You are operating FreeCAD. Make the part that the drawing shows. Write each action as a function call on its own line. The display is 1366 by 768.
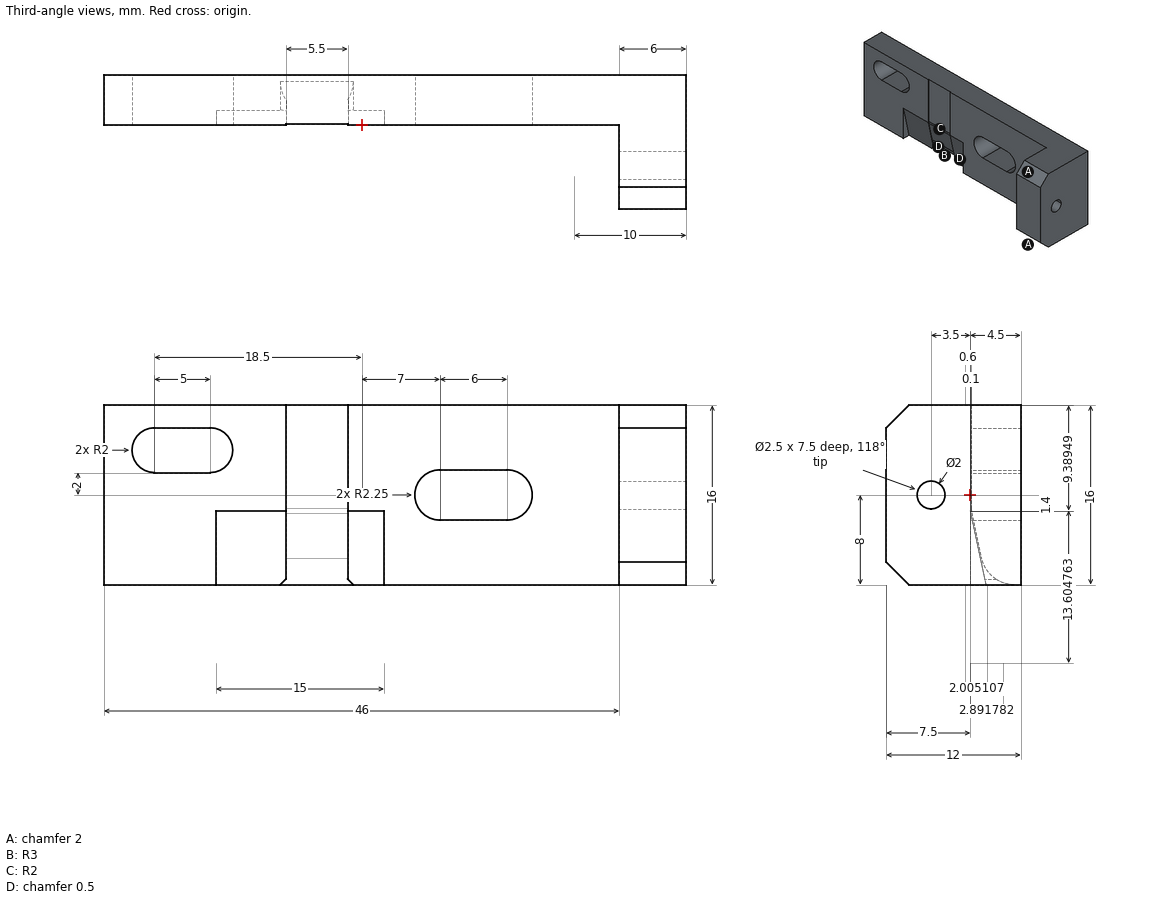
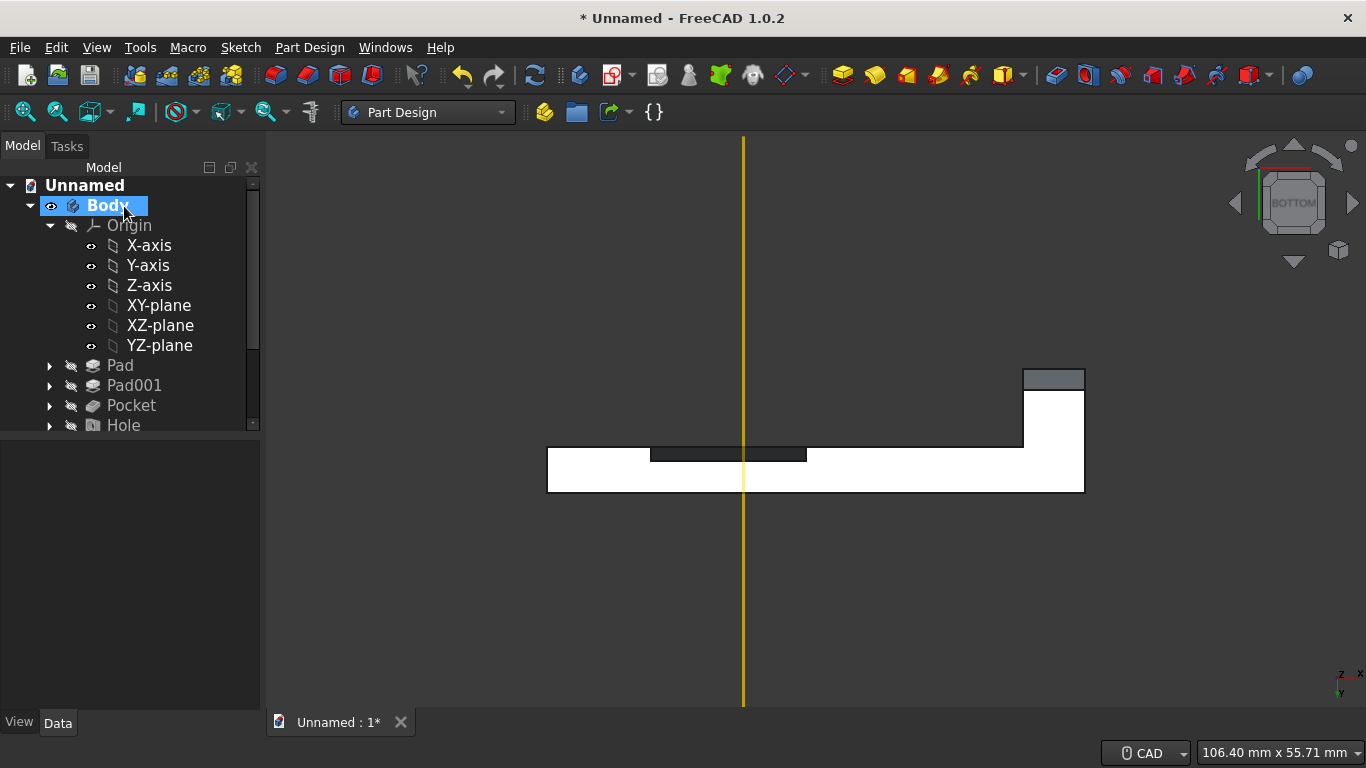
scroll(100, 301, down, 3)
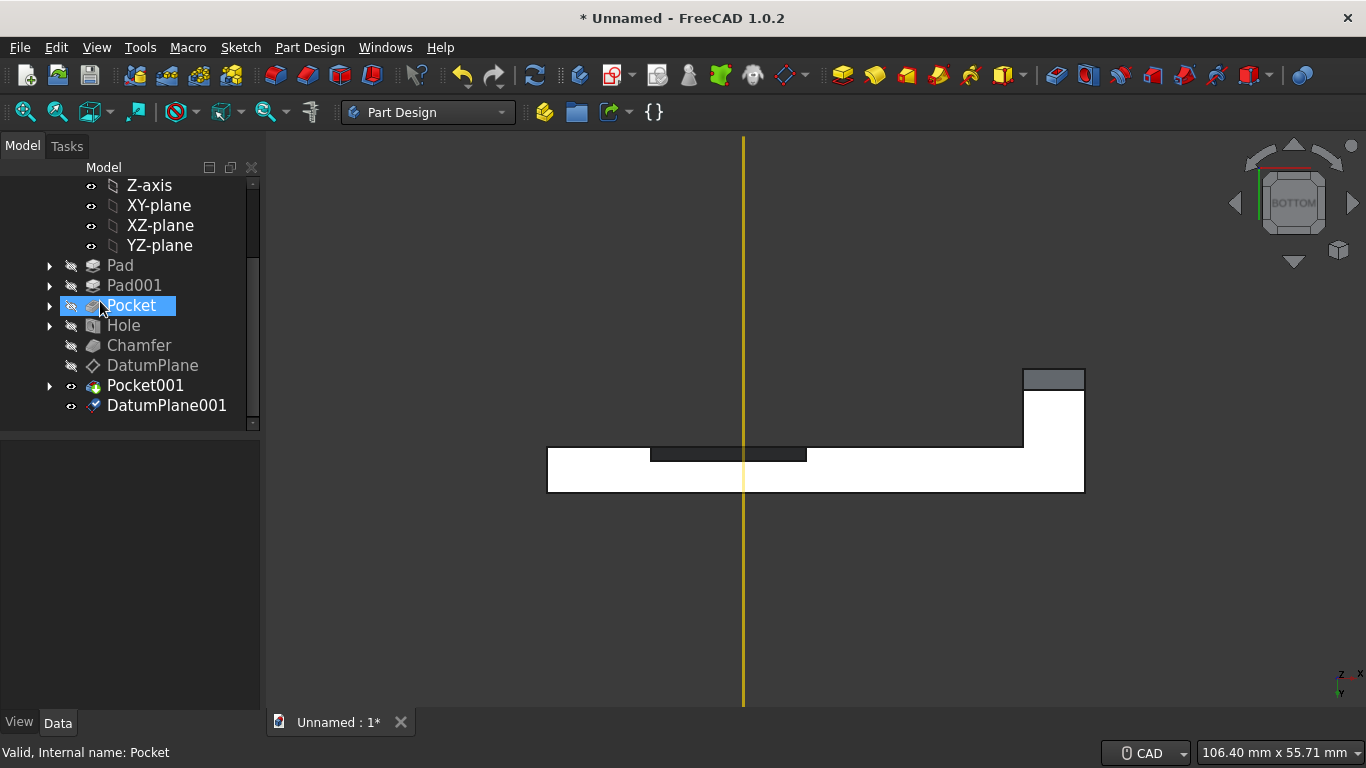
click(116, 406)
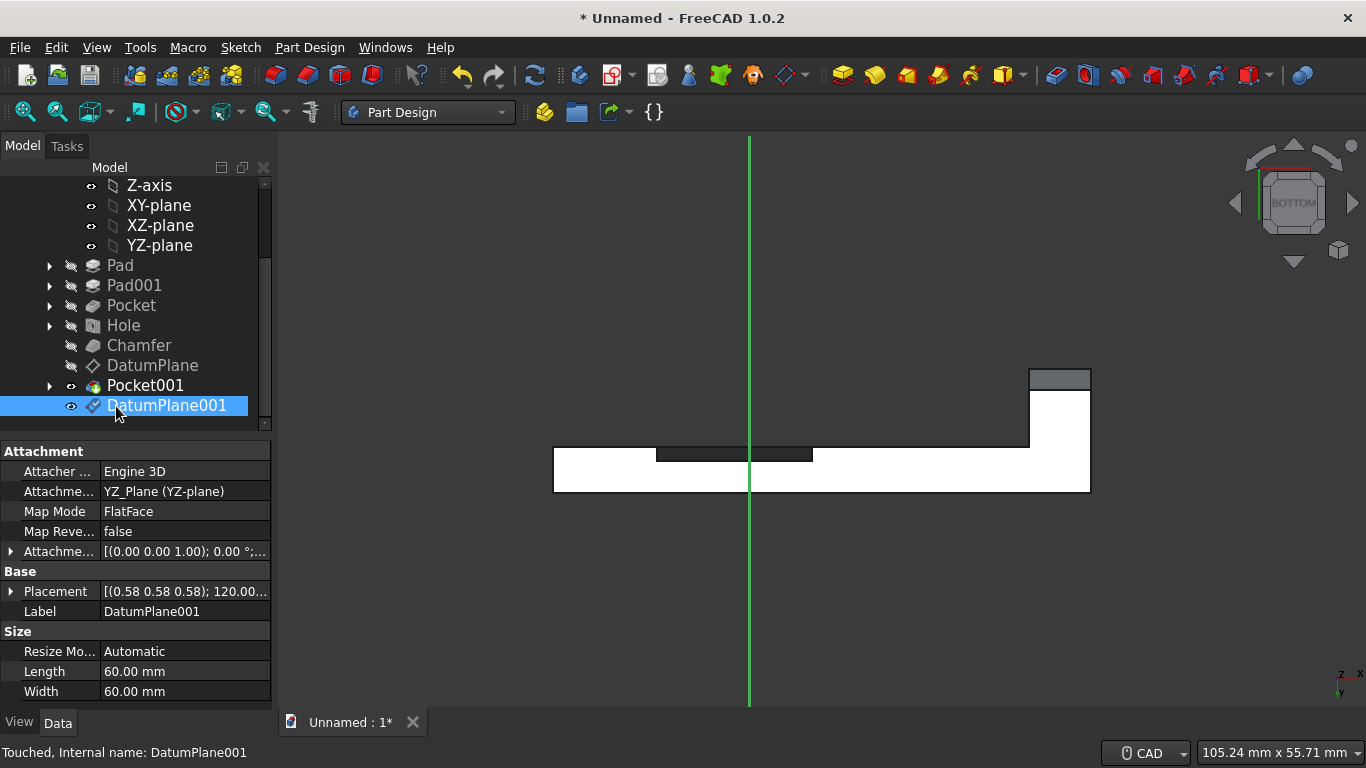
click(612, 76)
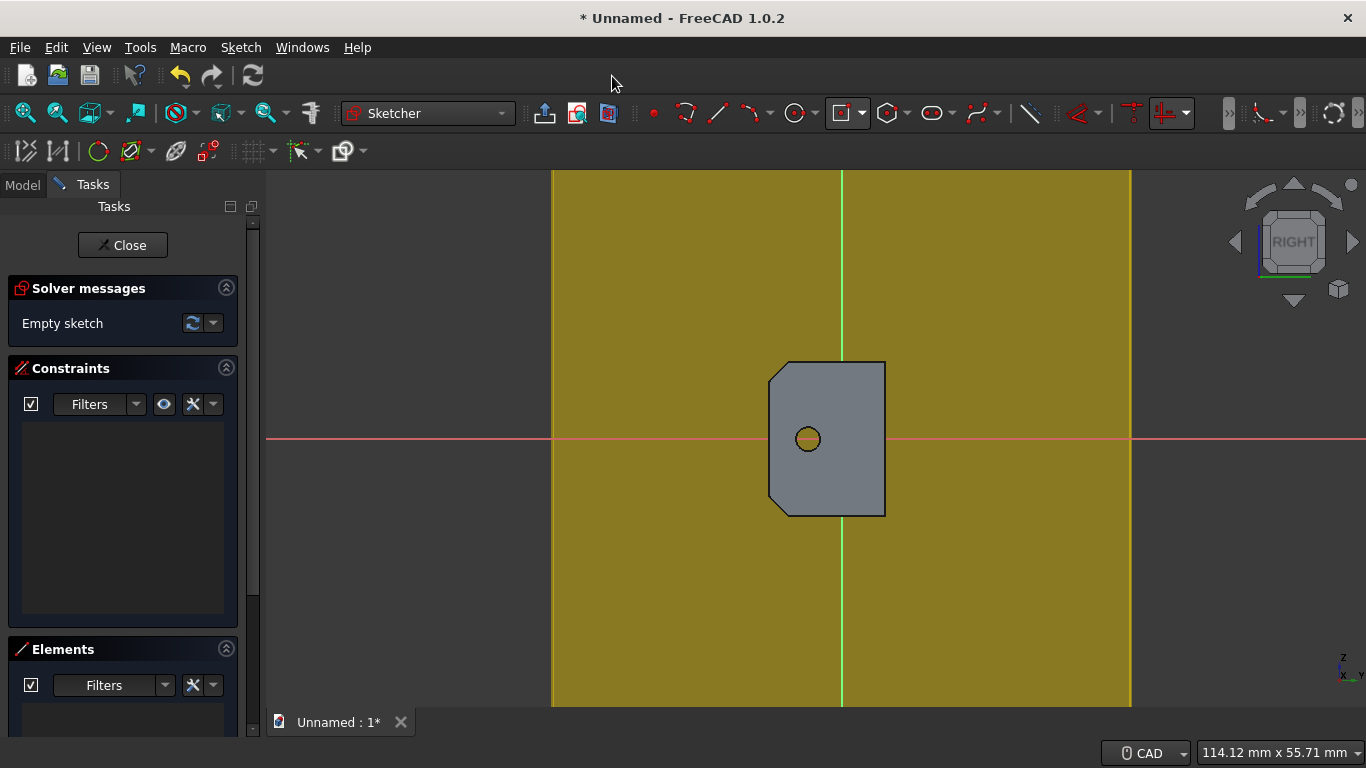
click(610, 114)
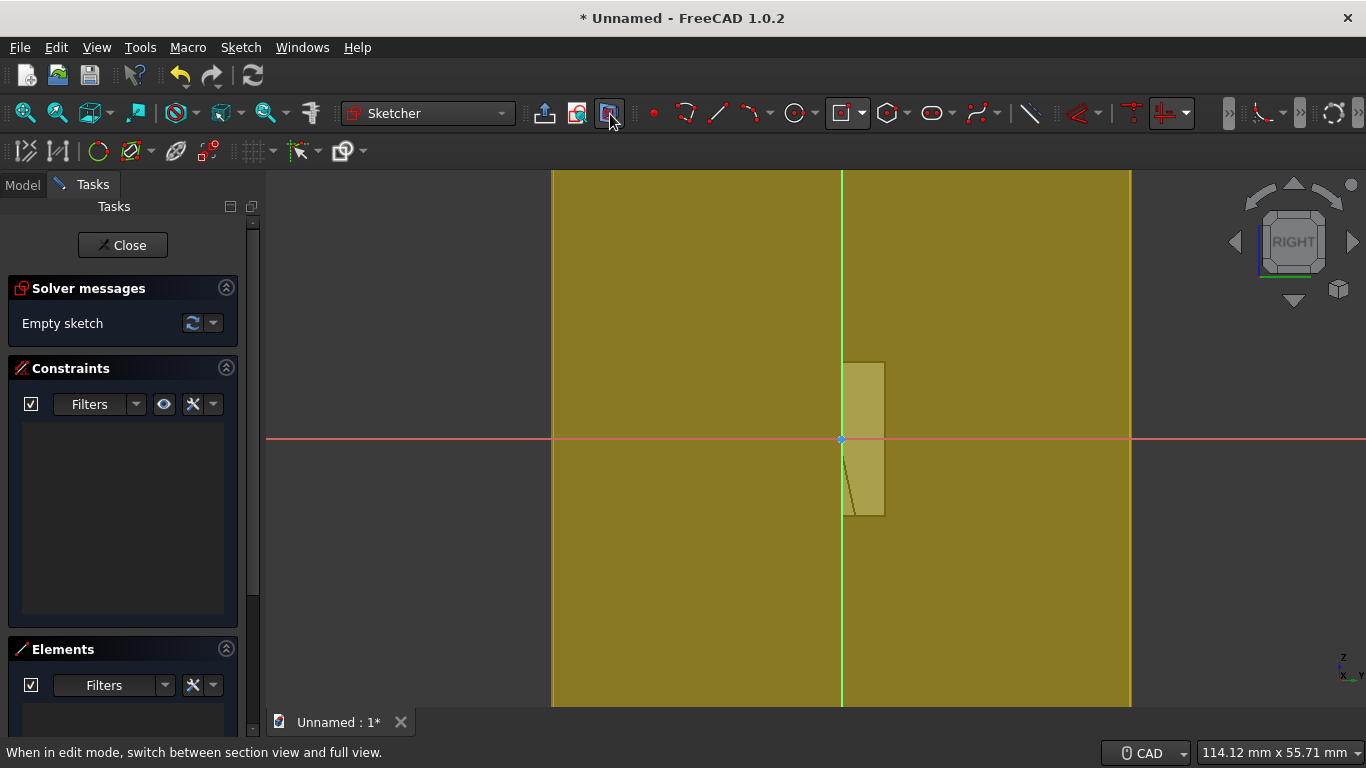
scroll(928, 440, up, 4)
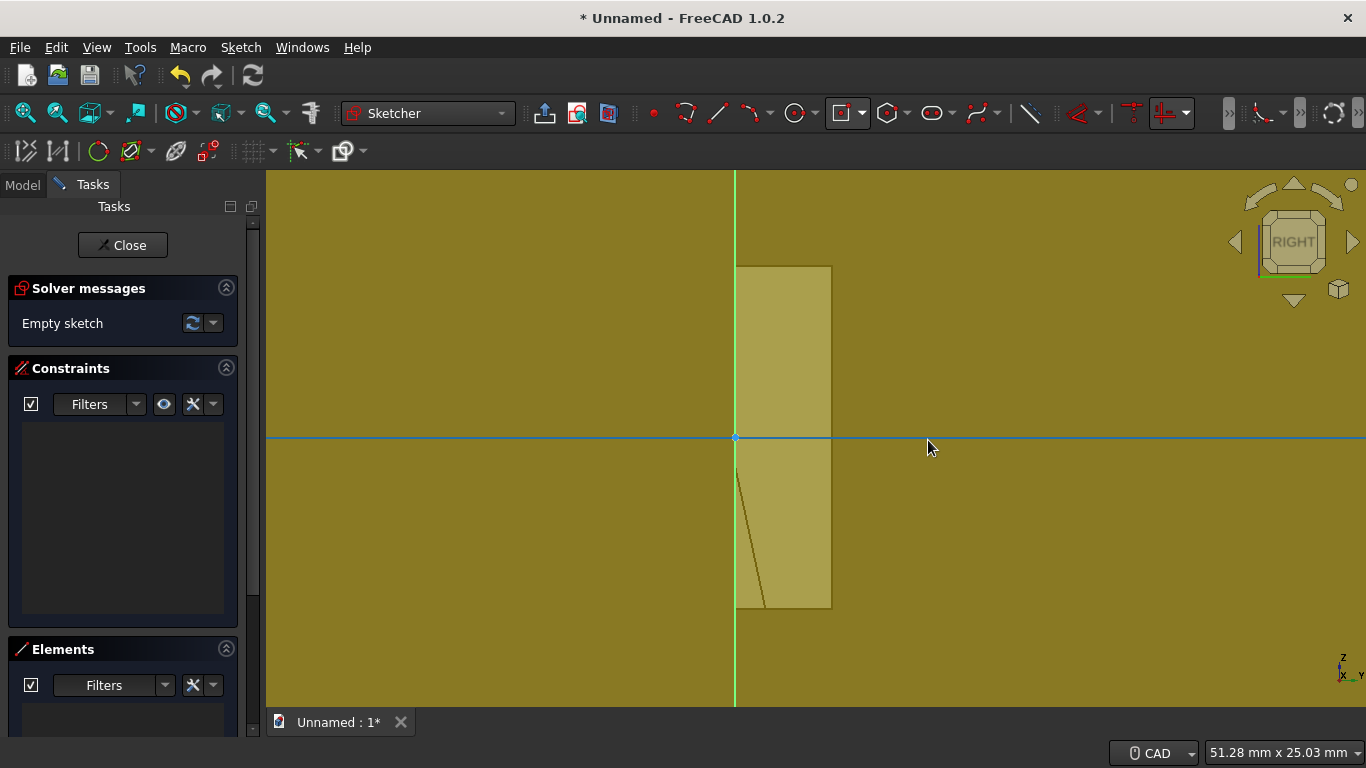
key(g)
key(m)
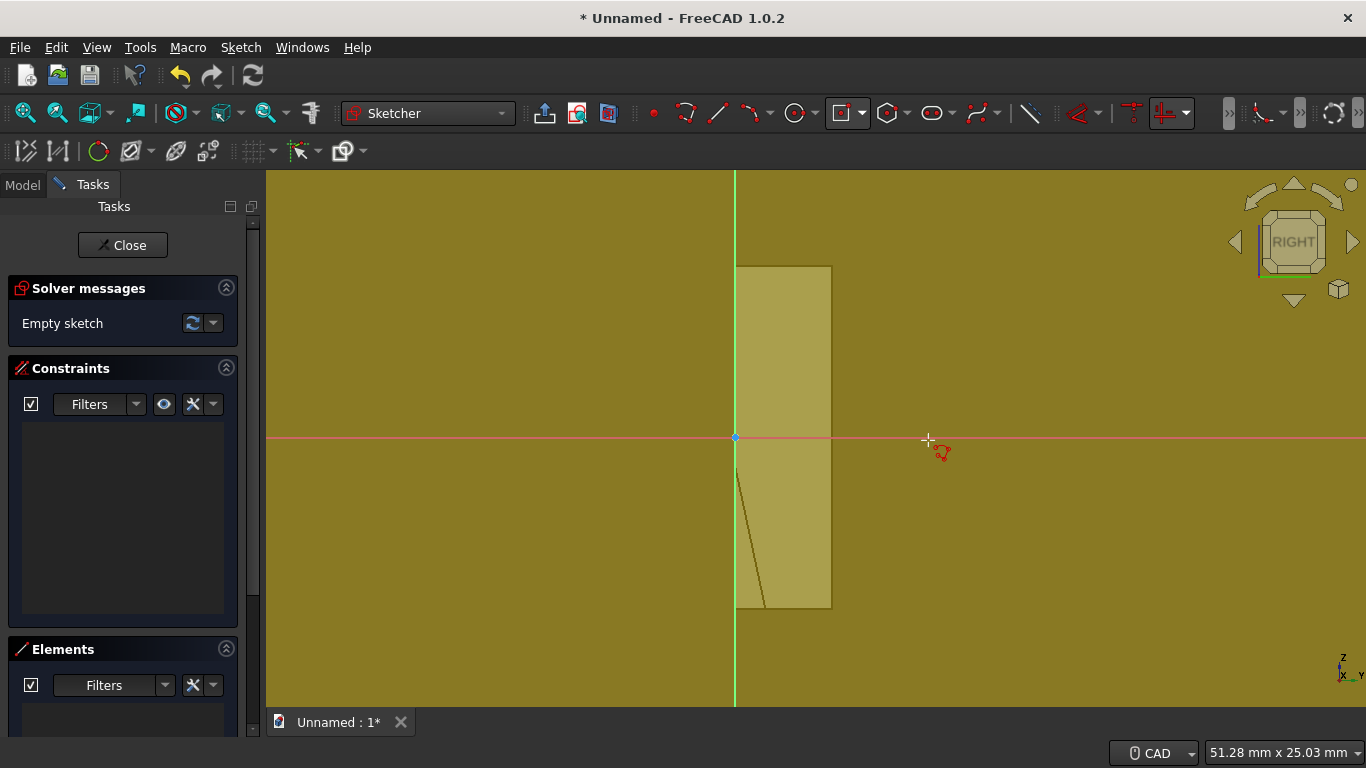
scroll(738, 467, up, 11)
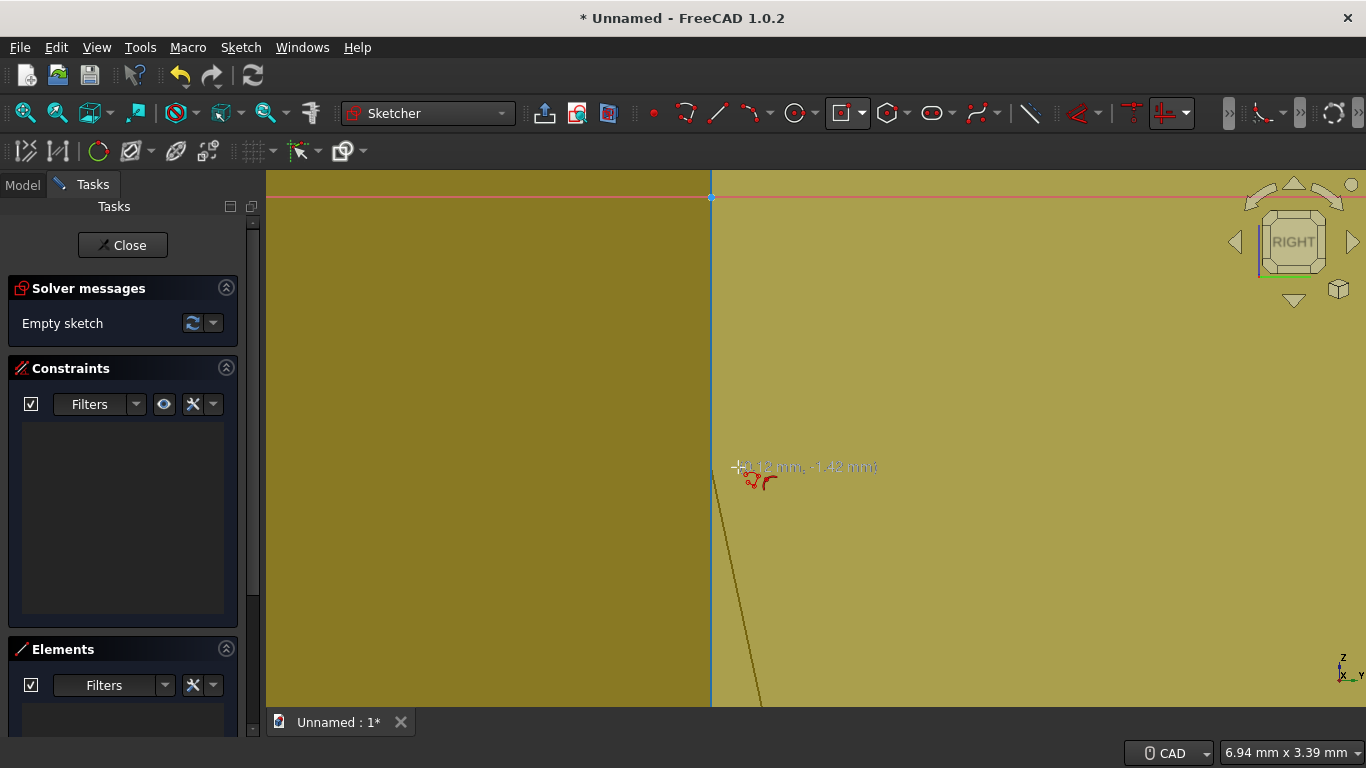
click(730, 466)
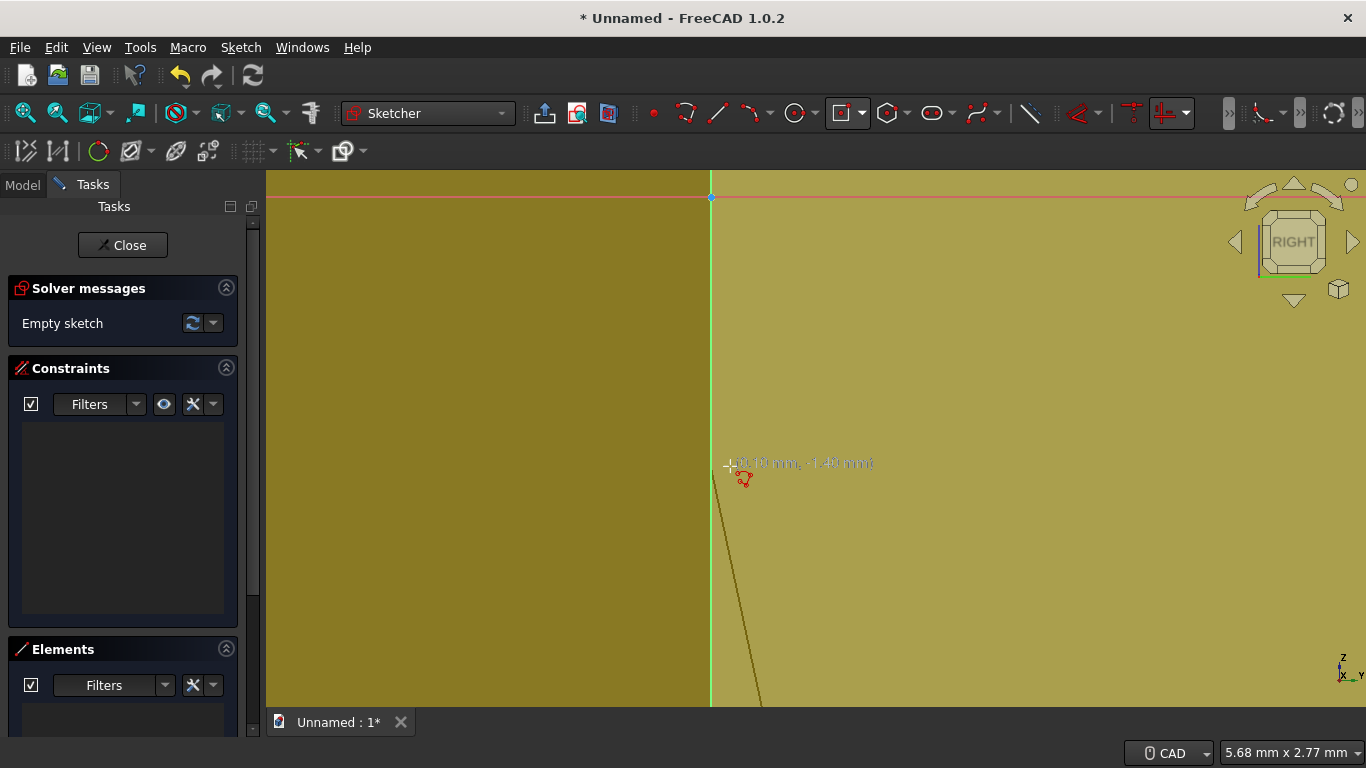
scroll(740, 469, down, 11)